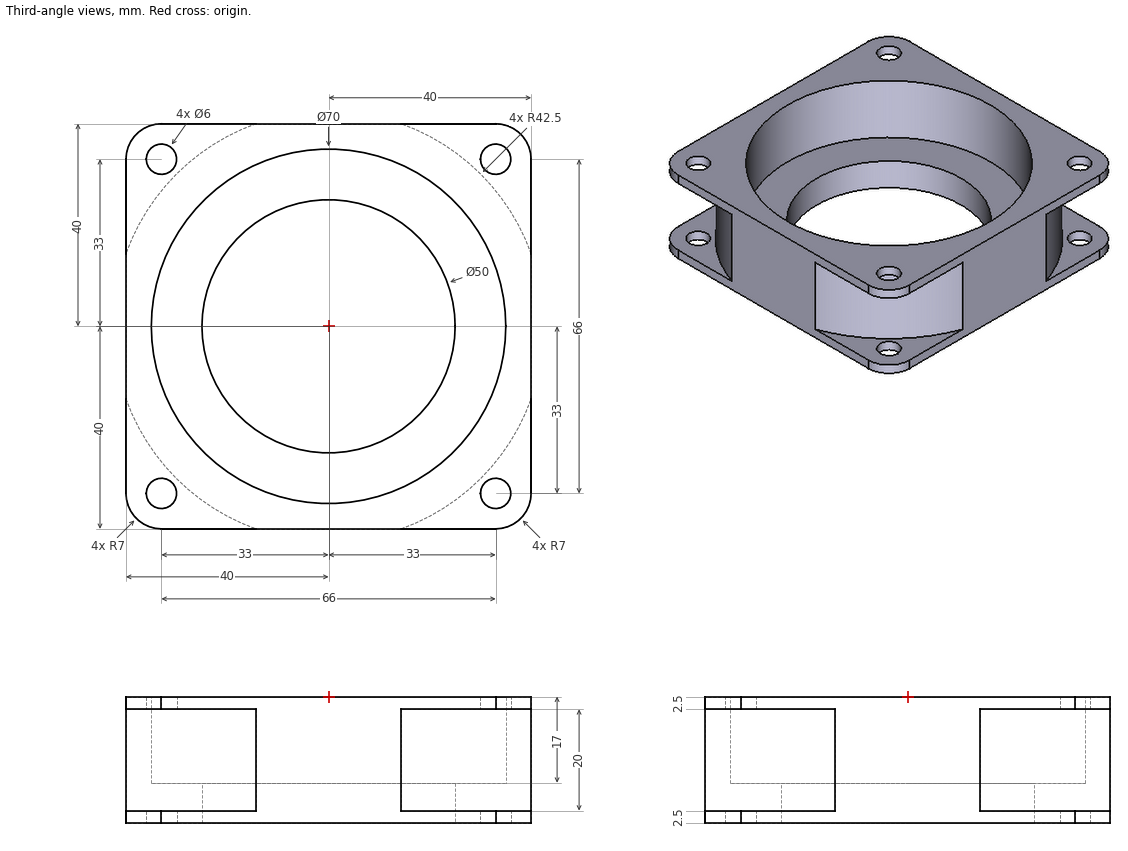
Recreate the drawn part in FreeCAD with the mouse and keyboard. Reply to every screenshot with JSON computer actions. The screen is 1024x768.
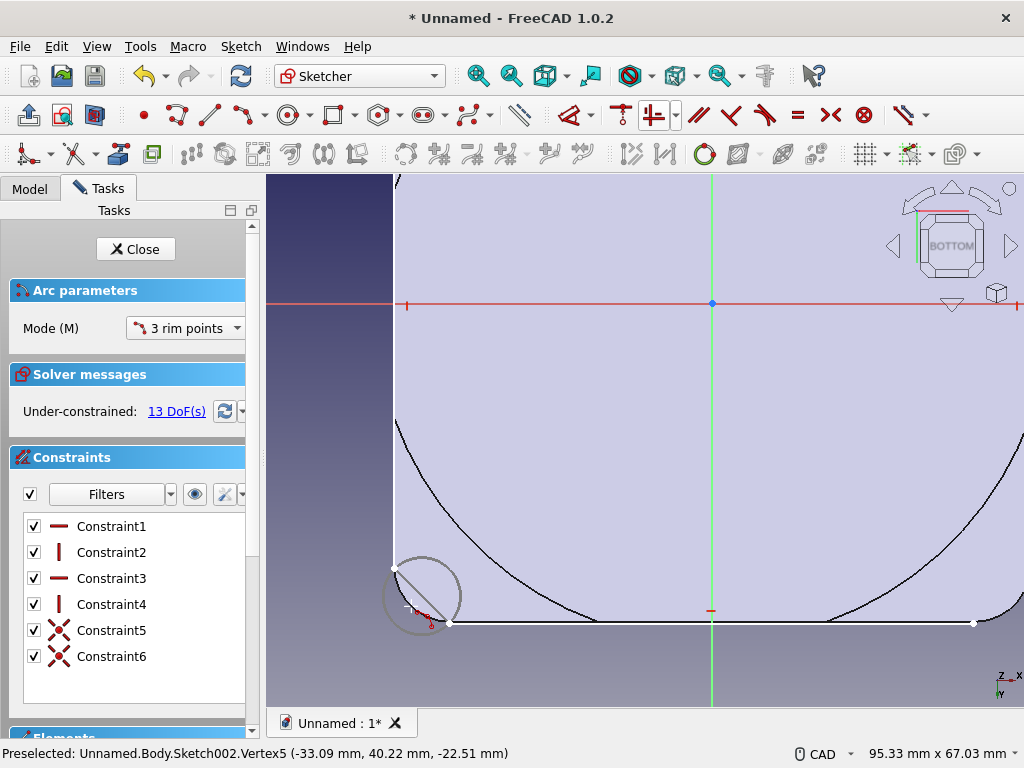
{"action": "left_click", "coordinate": [410, 606]}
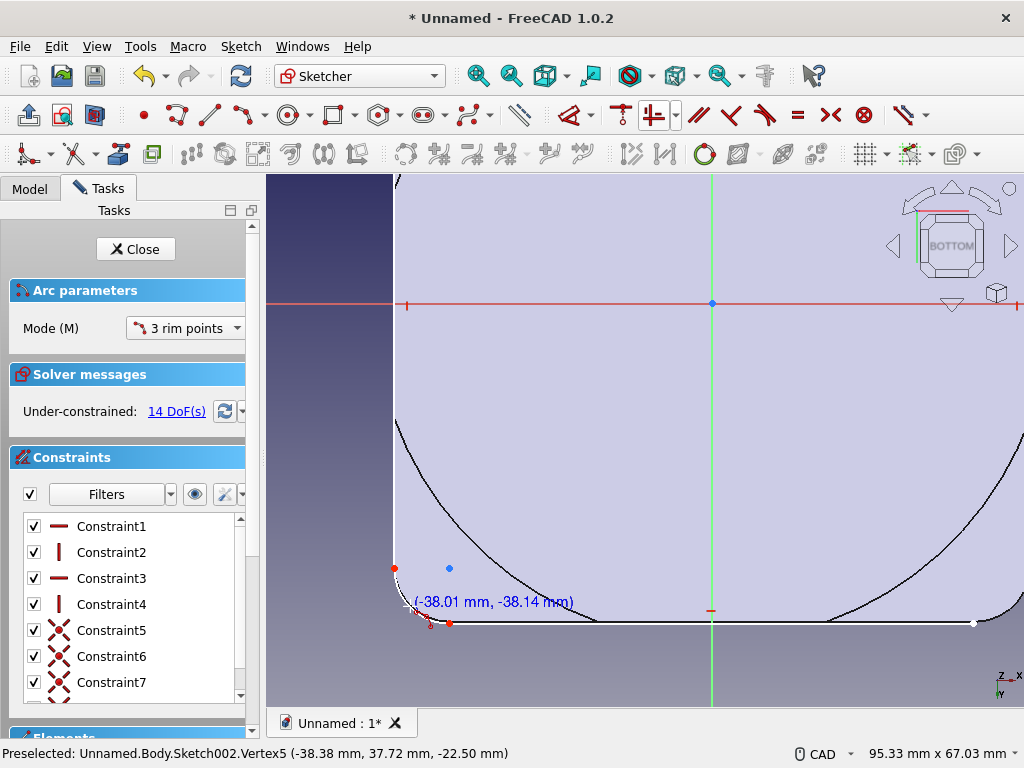
{"action": "scroll", "coordinate": [411, 607], "scroll_direction": "down", "scroll_amount": 3}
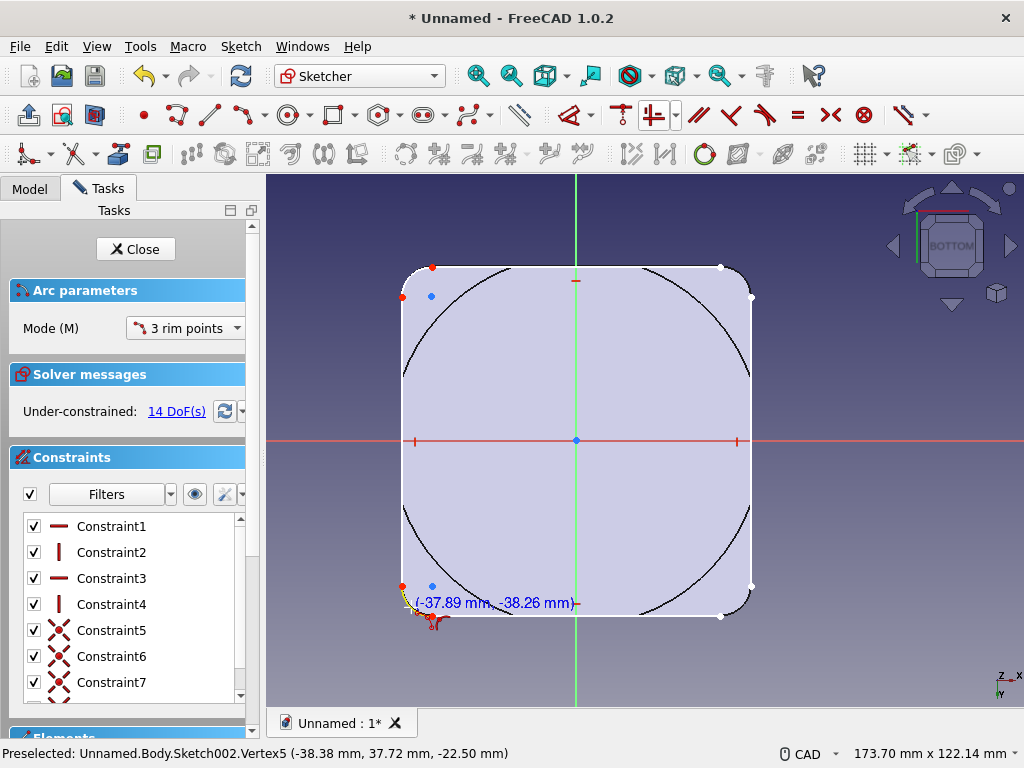
{"action": "left_click", "coordinate": [720, 616]}
{"action": "left_click", "coordinate": [751, 586]}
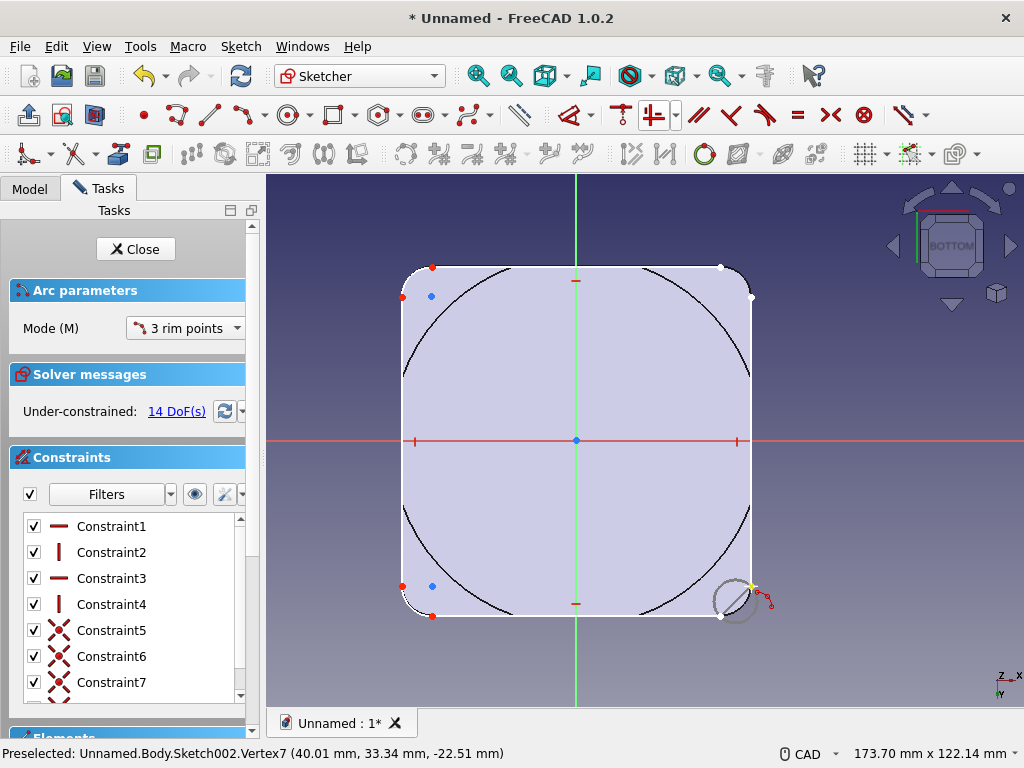
{"action": "scroll", "coordinate": [742, 607], "scroll_direction": "up", "scroll_amount": 3}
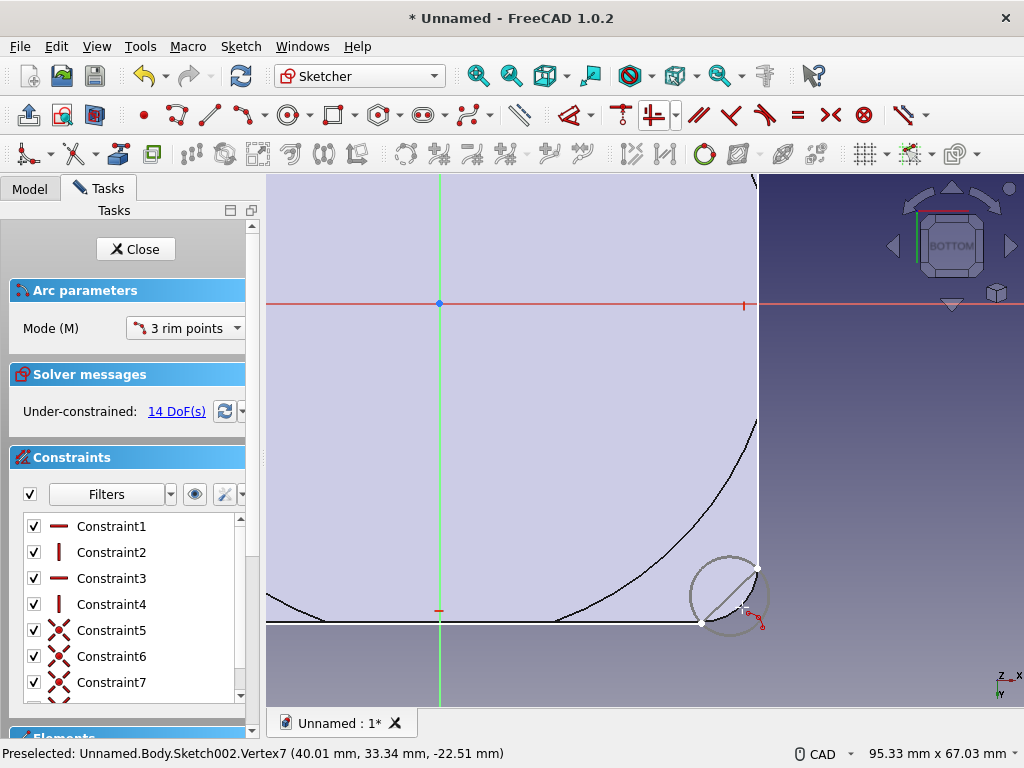
{"action": "left_click", "coordinate": [742, 606]}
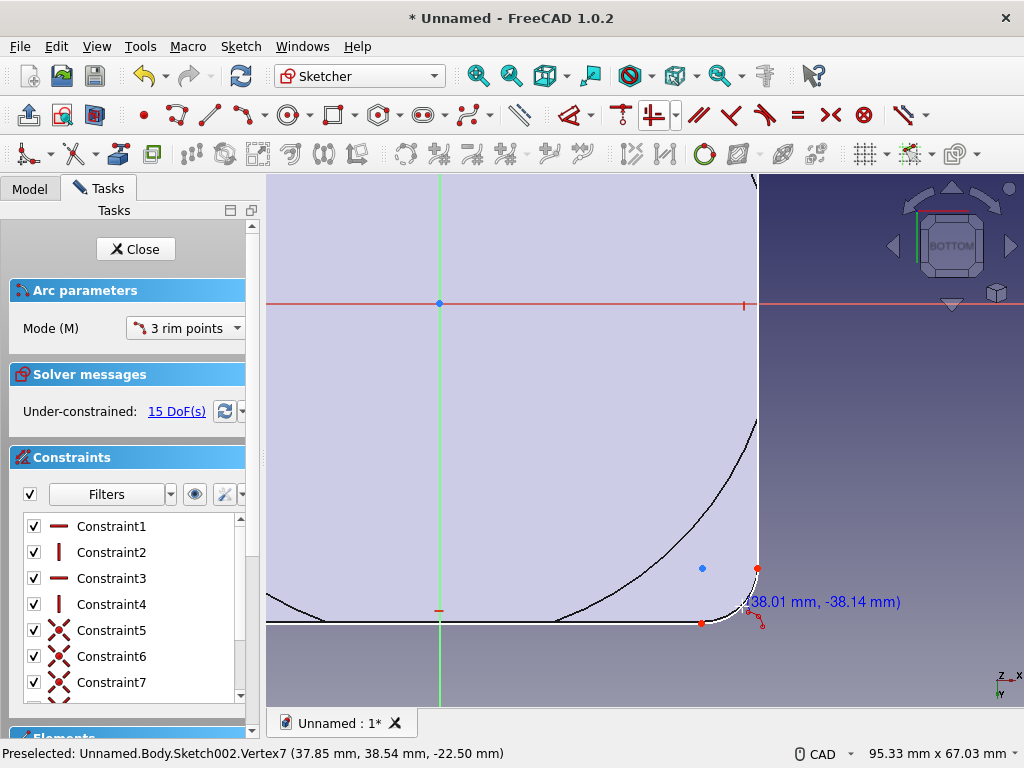
{"action": "scroll", "coordinate": [743, 607], "scroll_direction": "down", "scroll_amount": 3}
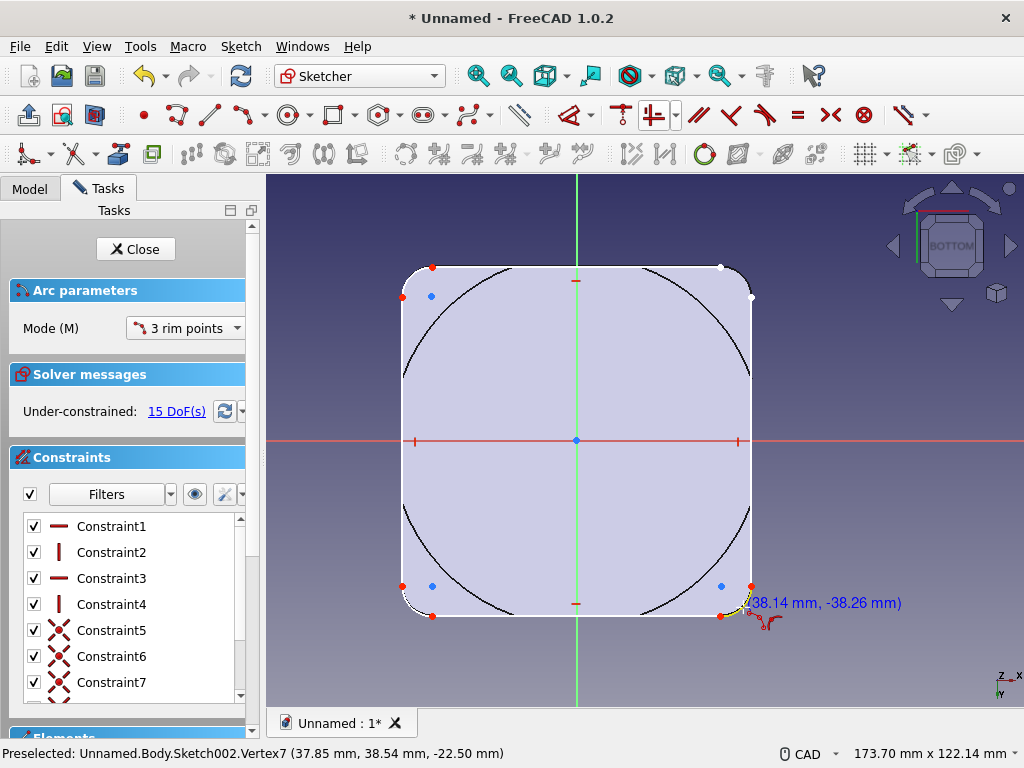
{"action": "left_click", "coordinate": [751, 297]}
{"action": "left_click", "coordinate": [720, 267]}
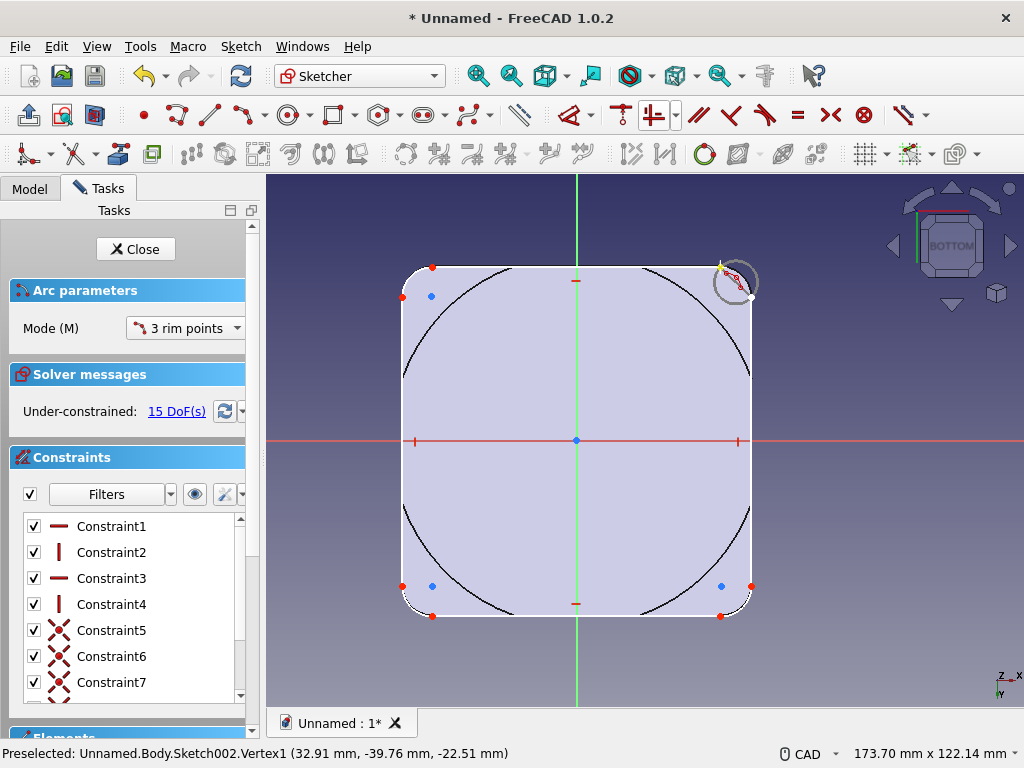
{"action": "scroll", "coordinate": [742, 275], "scroll_direction": "up", "scroll_amount": 3}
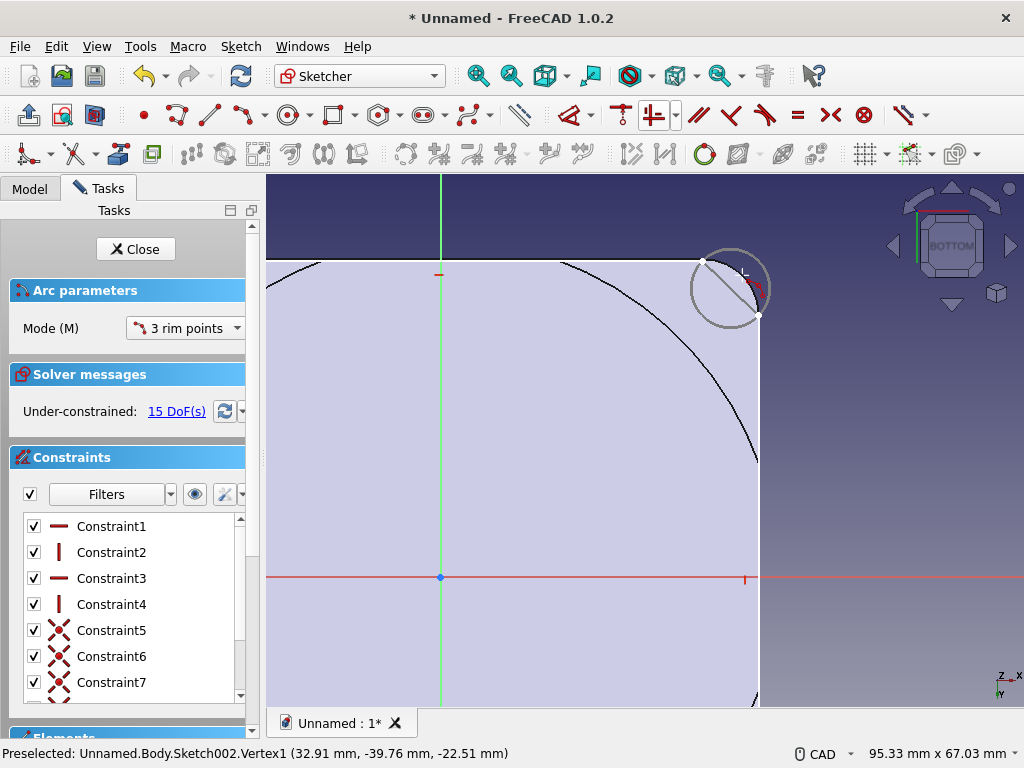
{"action": "left_click", "coordinate": [742, 275]}
{"action": "key", "text": "Escape"}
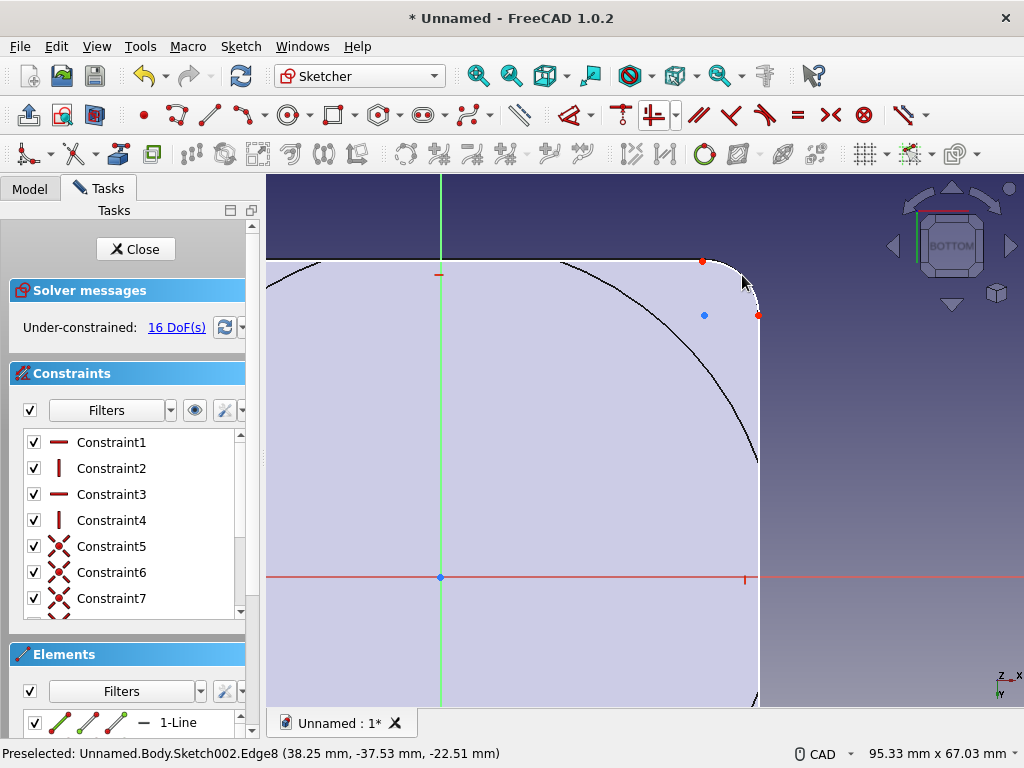
{"action": "left_click", "coordinate": [545, 261]}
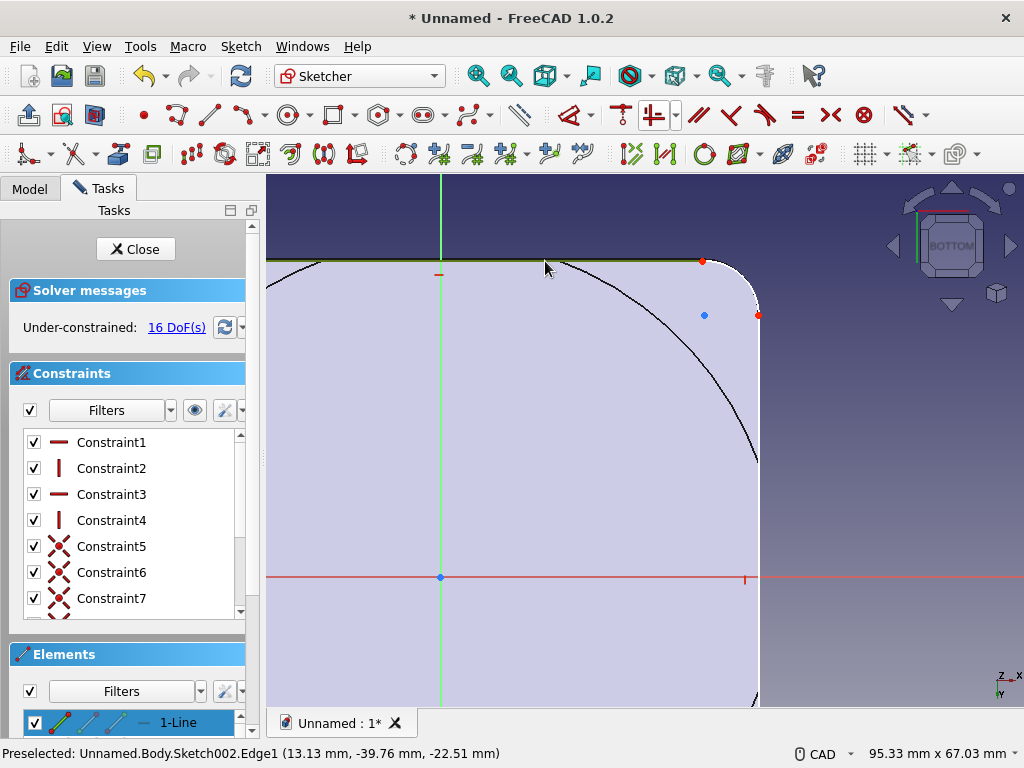
{"action": "scroll", "coordinate": [742, 274], "scroll_direction": "down", "scroll_amount": 3}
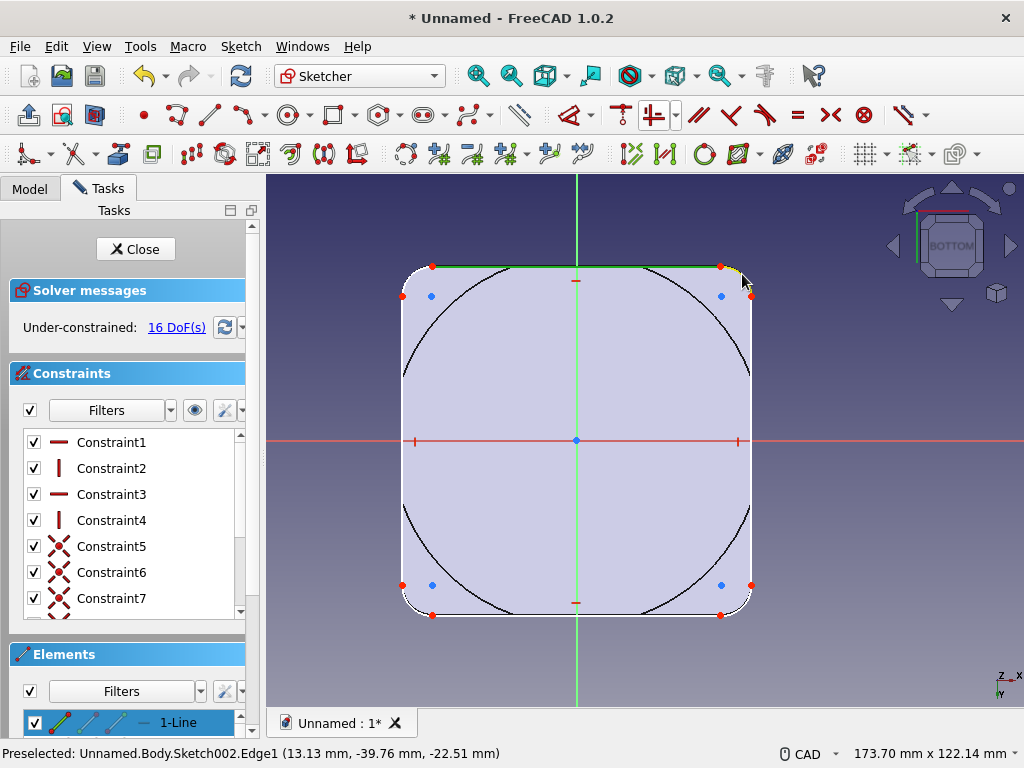
{"action": "left_click", "coordinate": [419, 270]}